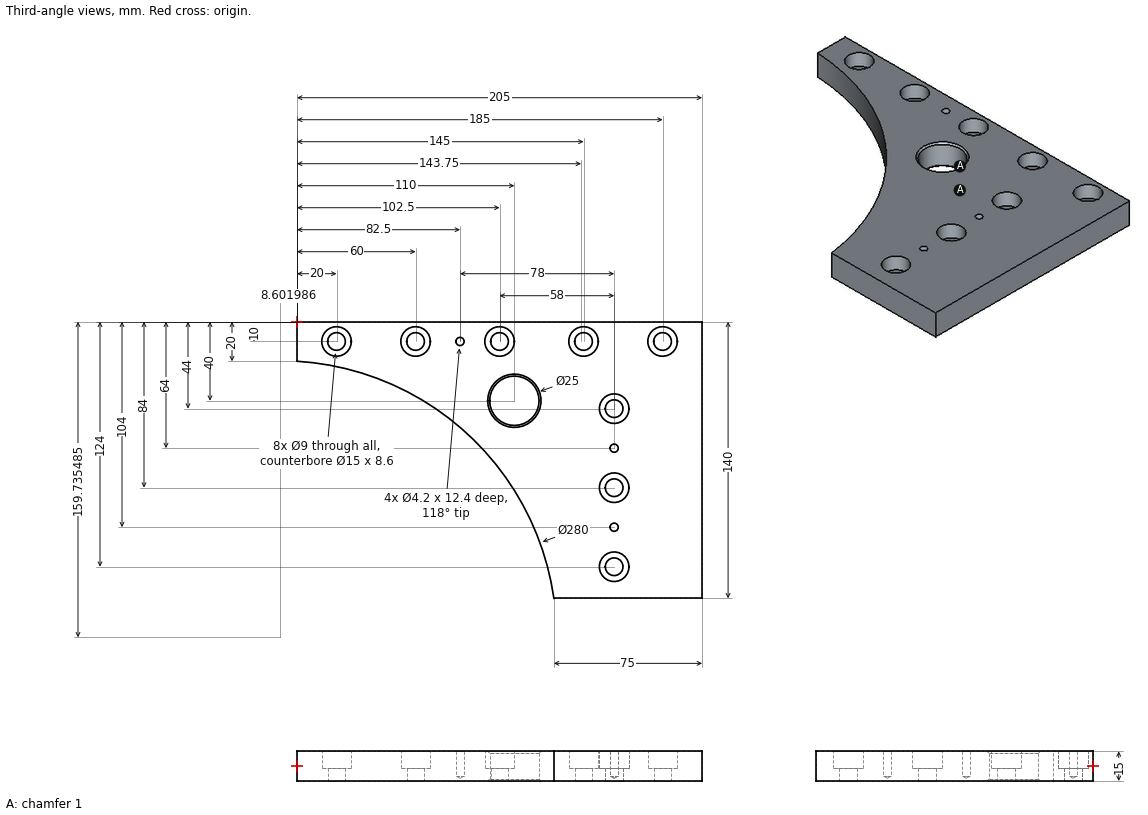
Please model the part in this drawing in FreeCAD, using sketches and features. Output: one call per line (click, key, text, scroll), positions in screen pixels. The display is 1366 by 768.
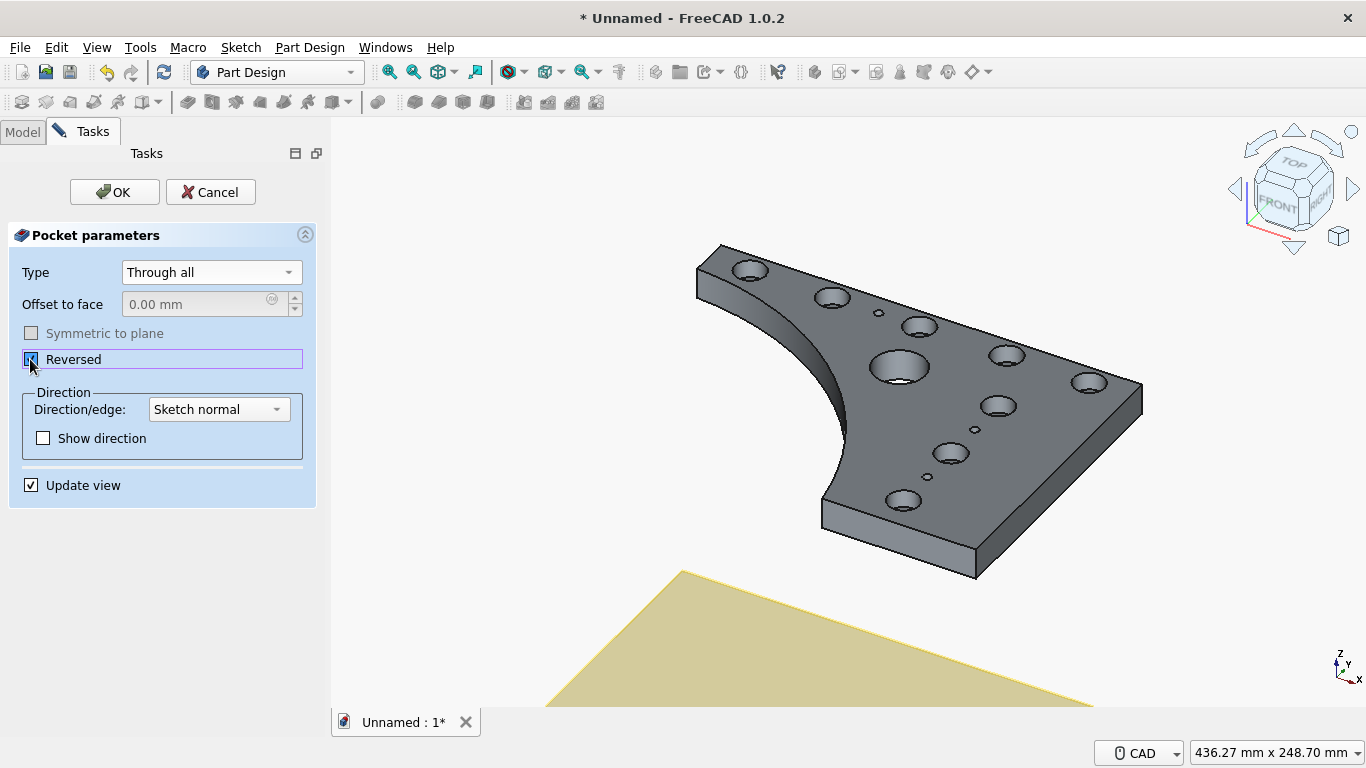
click(115, 192)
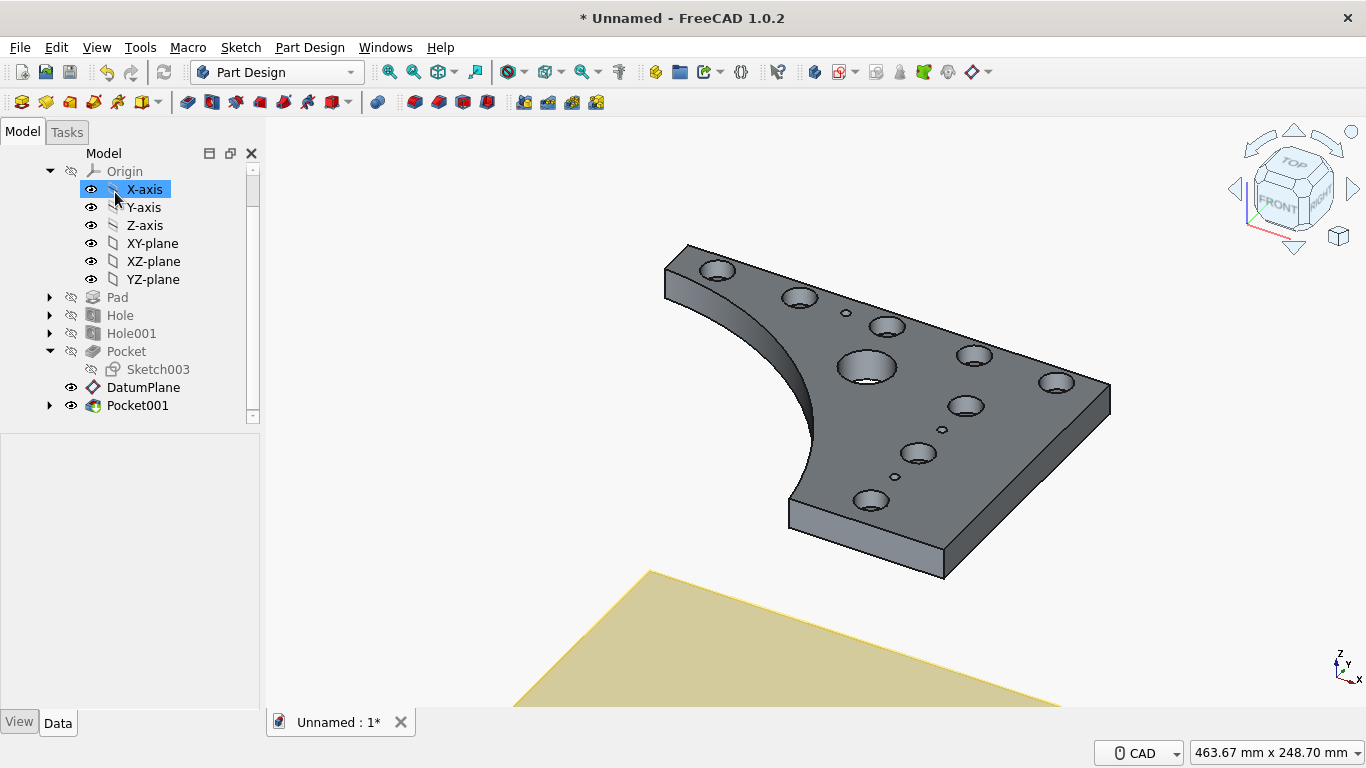
click(116, 387)
key(space)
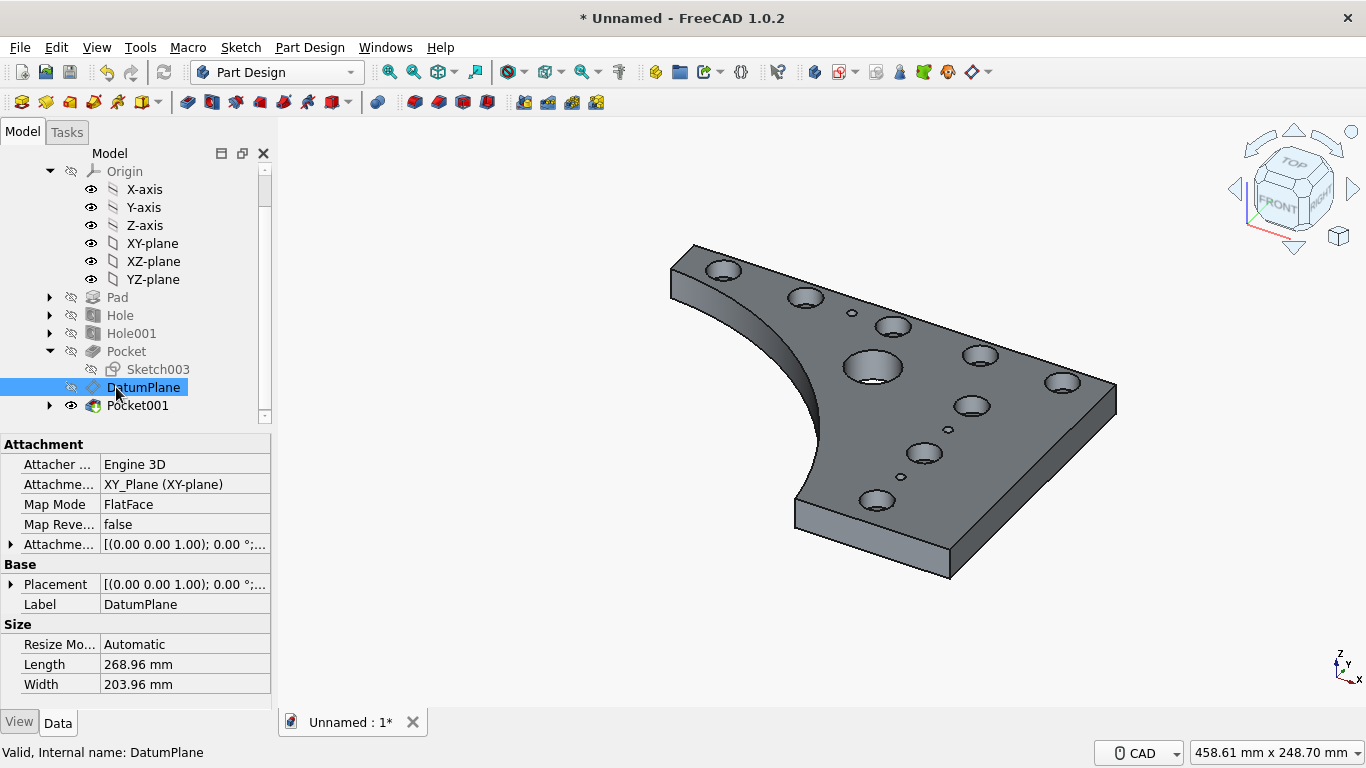
click(847, 358)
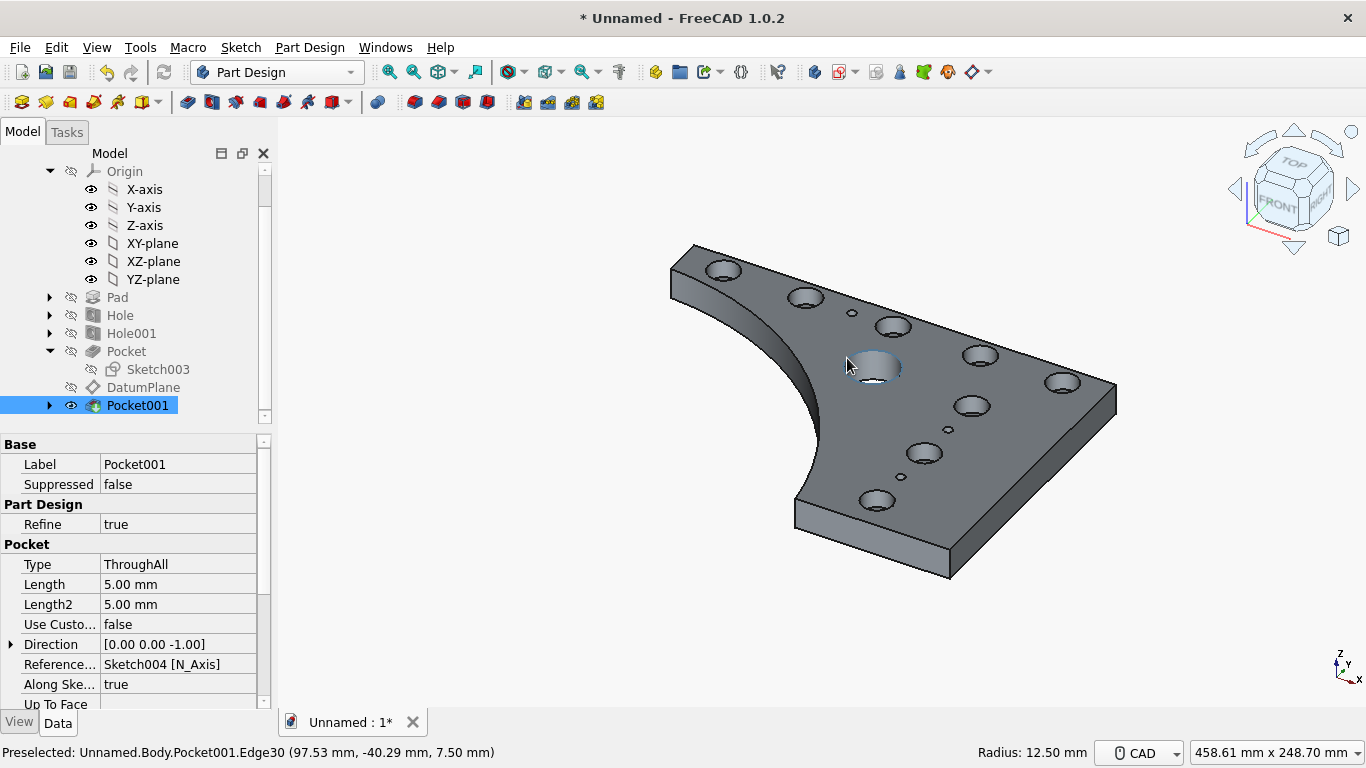
key(0)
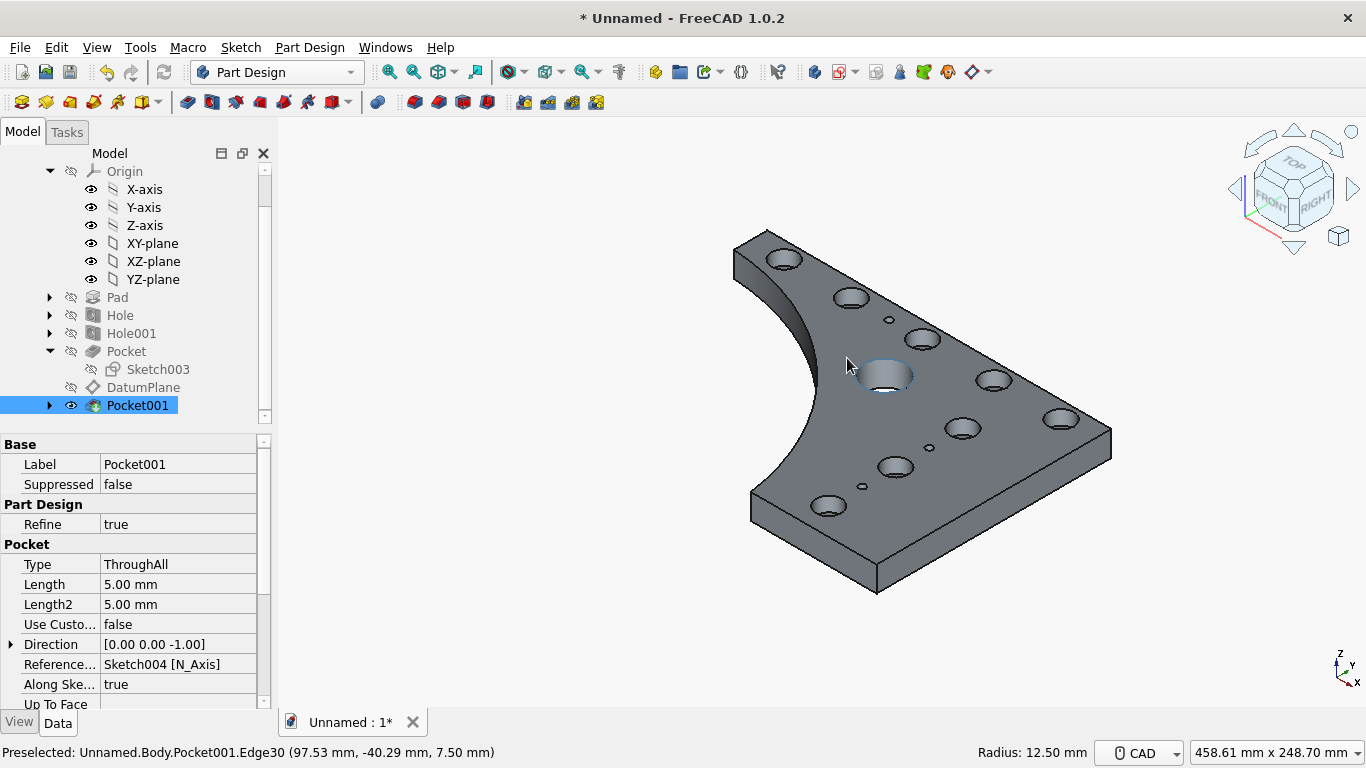
key(2)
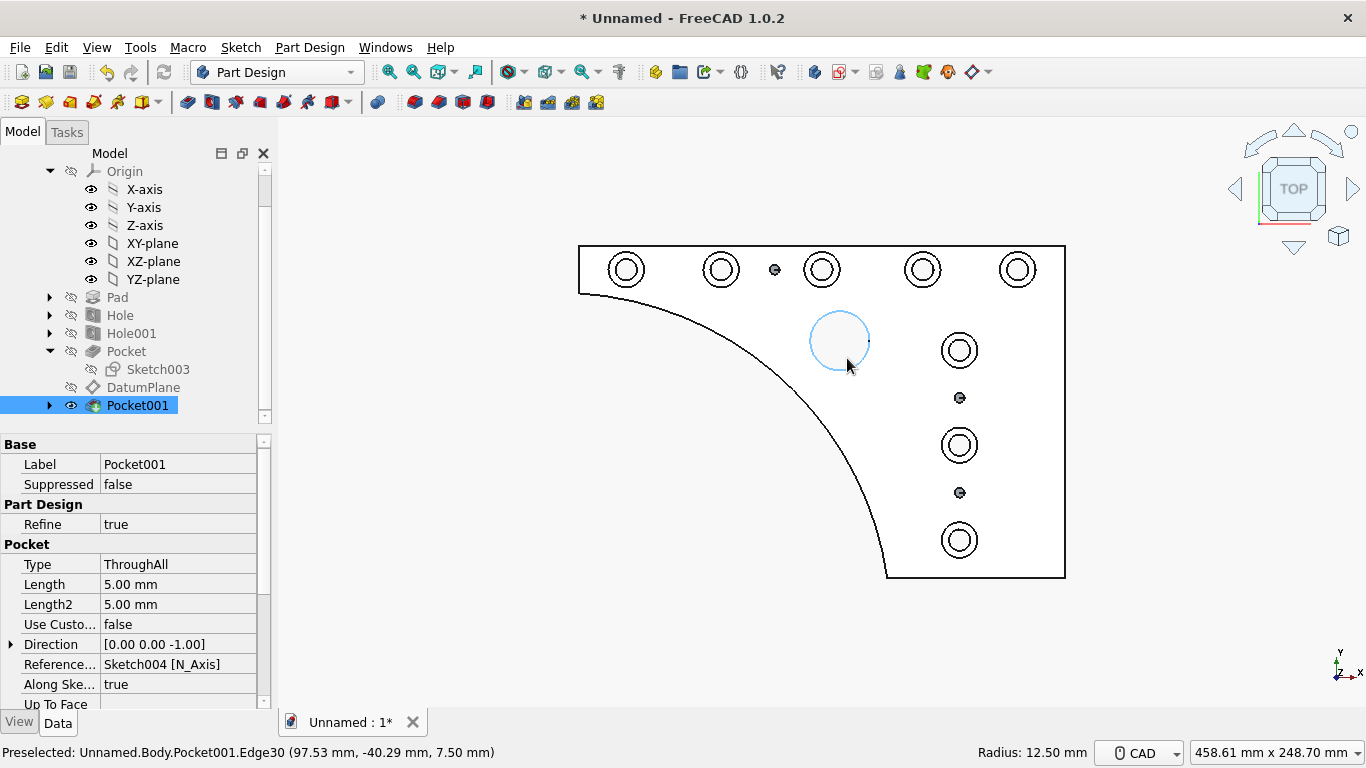
key(1)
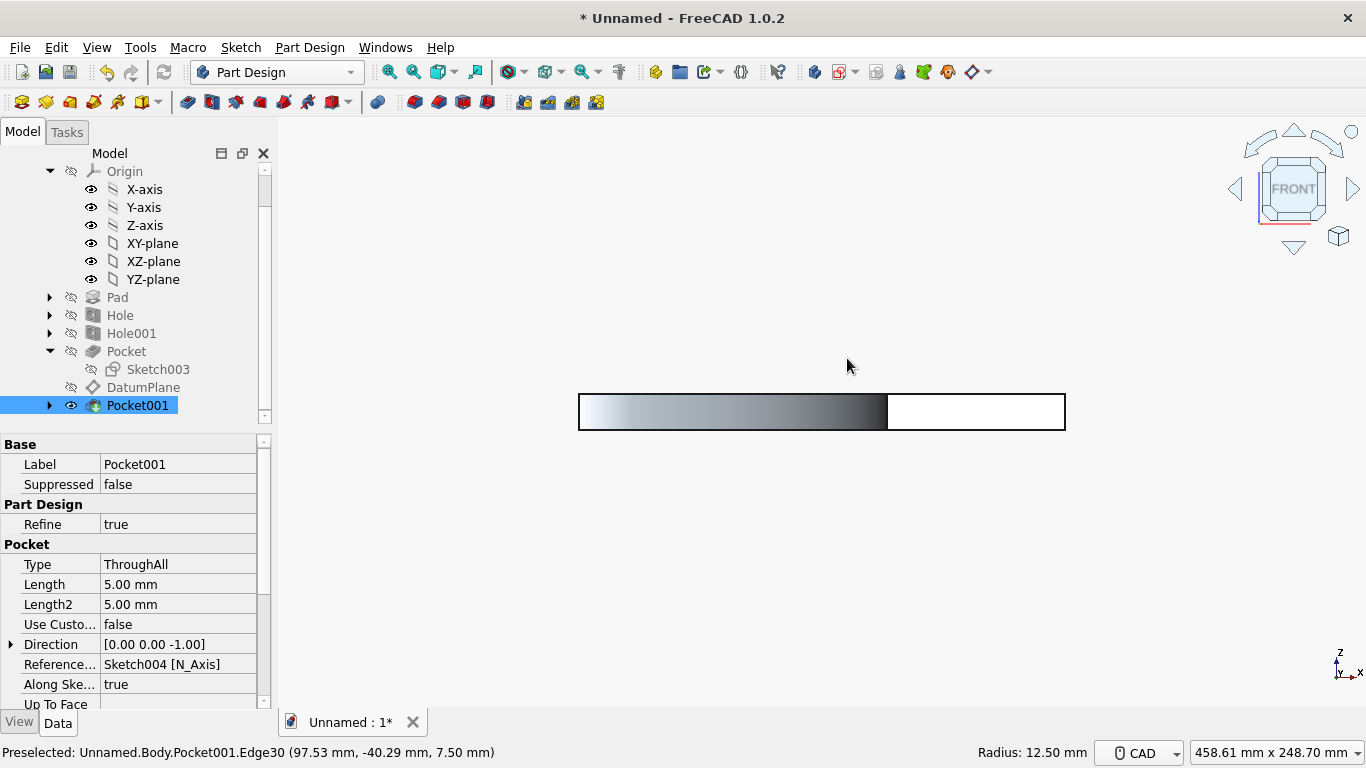
click(390, 72)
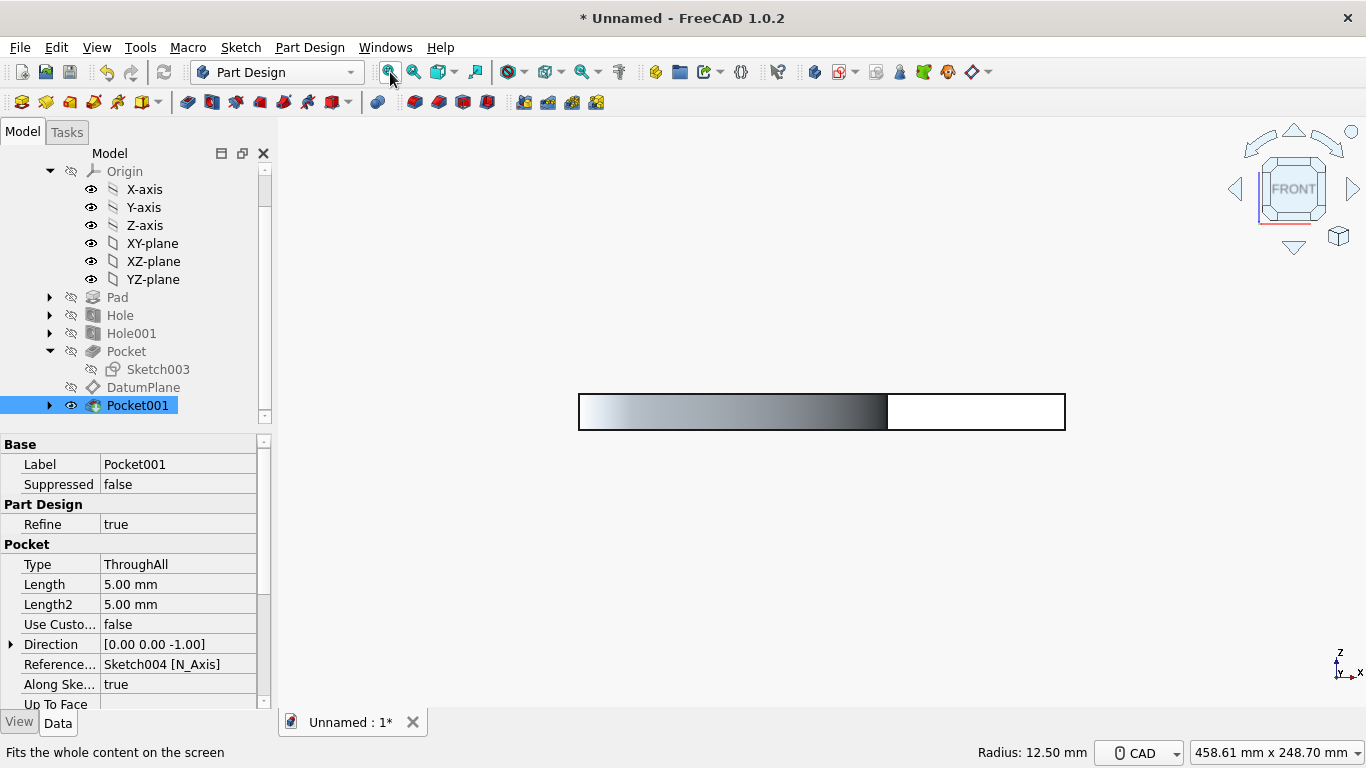
key(3)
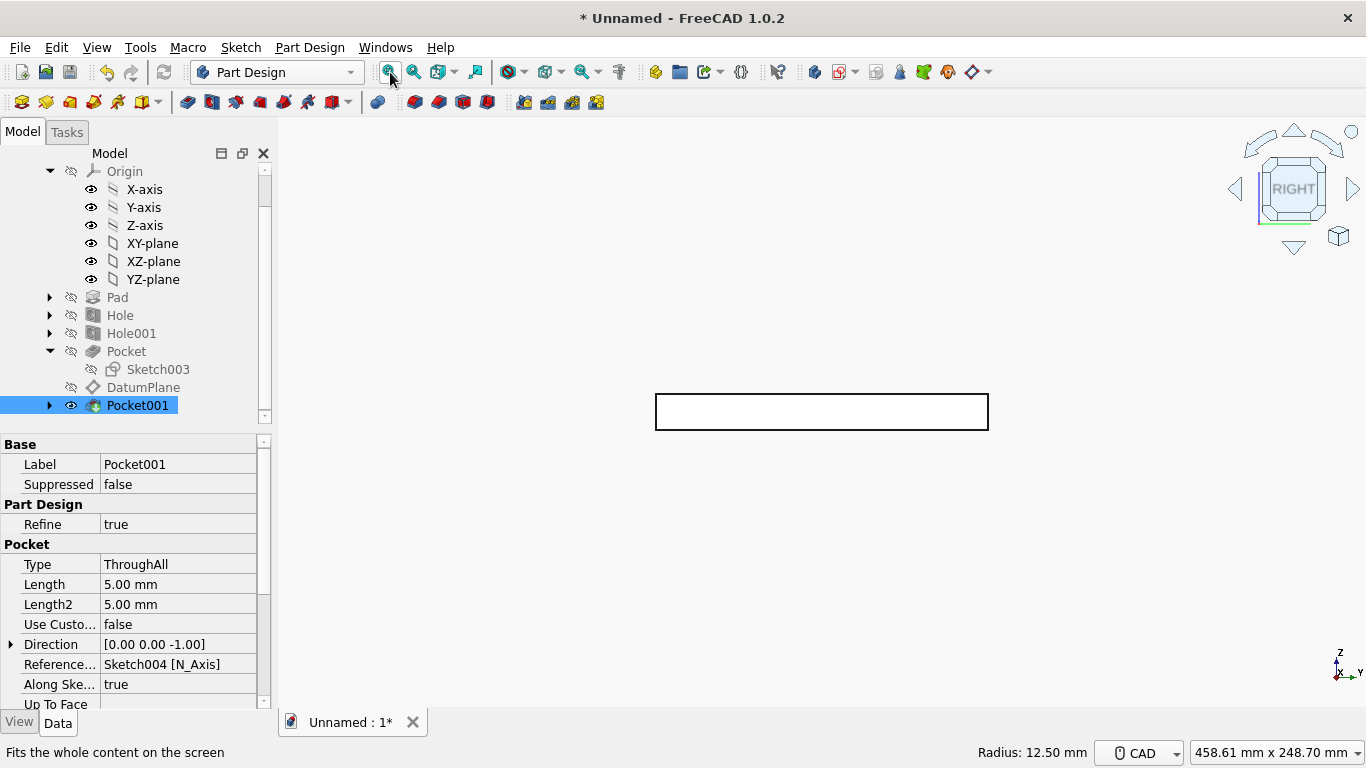
click(390, 72)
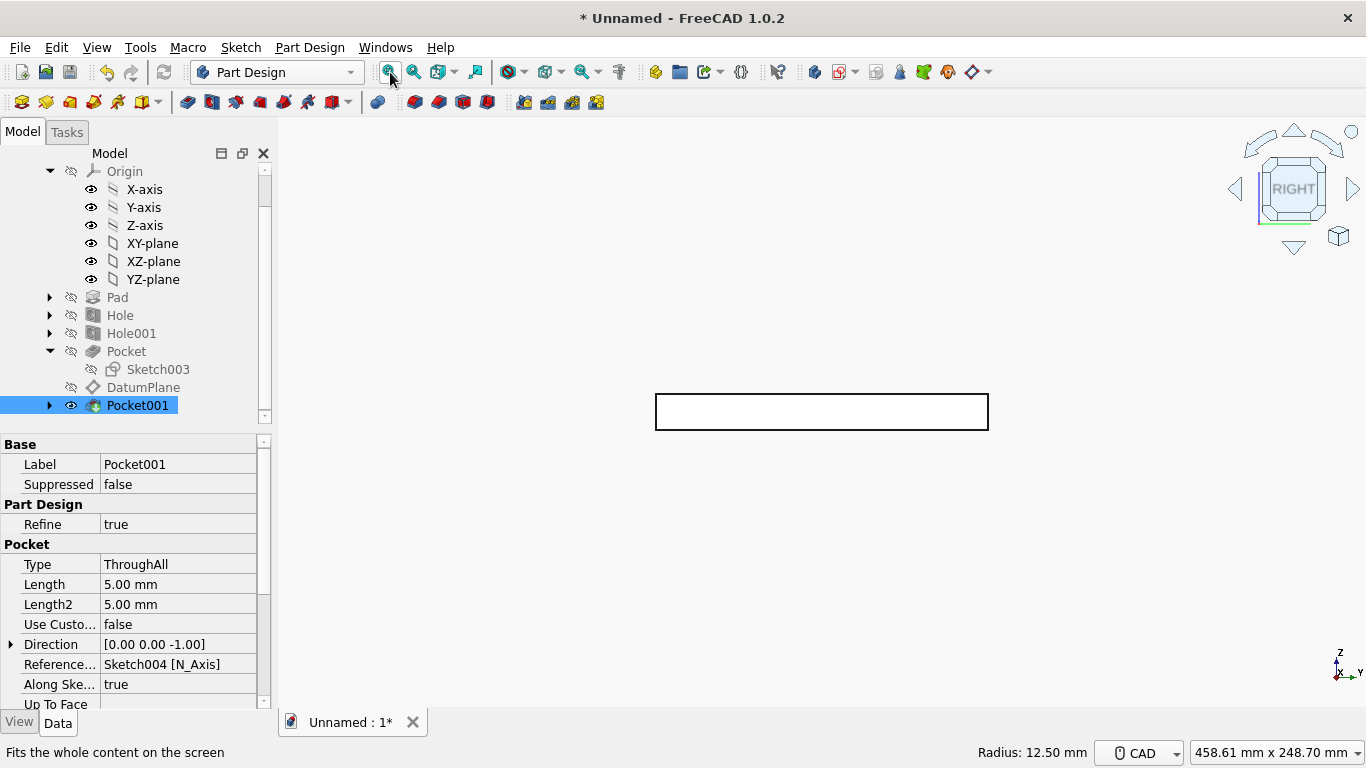
key(5)